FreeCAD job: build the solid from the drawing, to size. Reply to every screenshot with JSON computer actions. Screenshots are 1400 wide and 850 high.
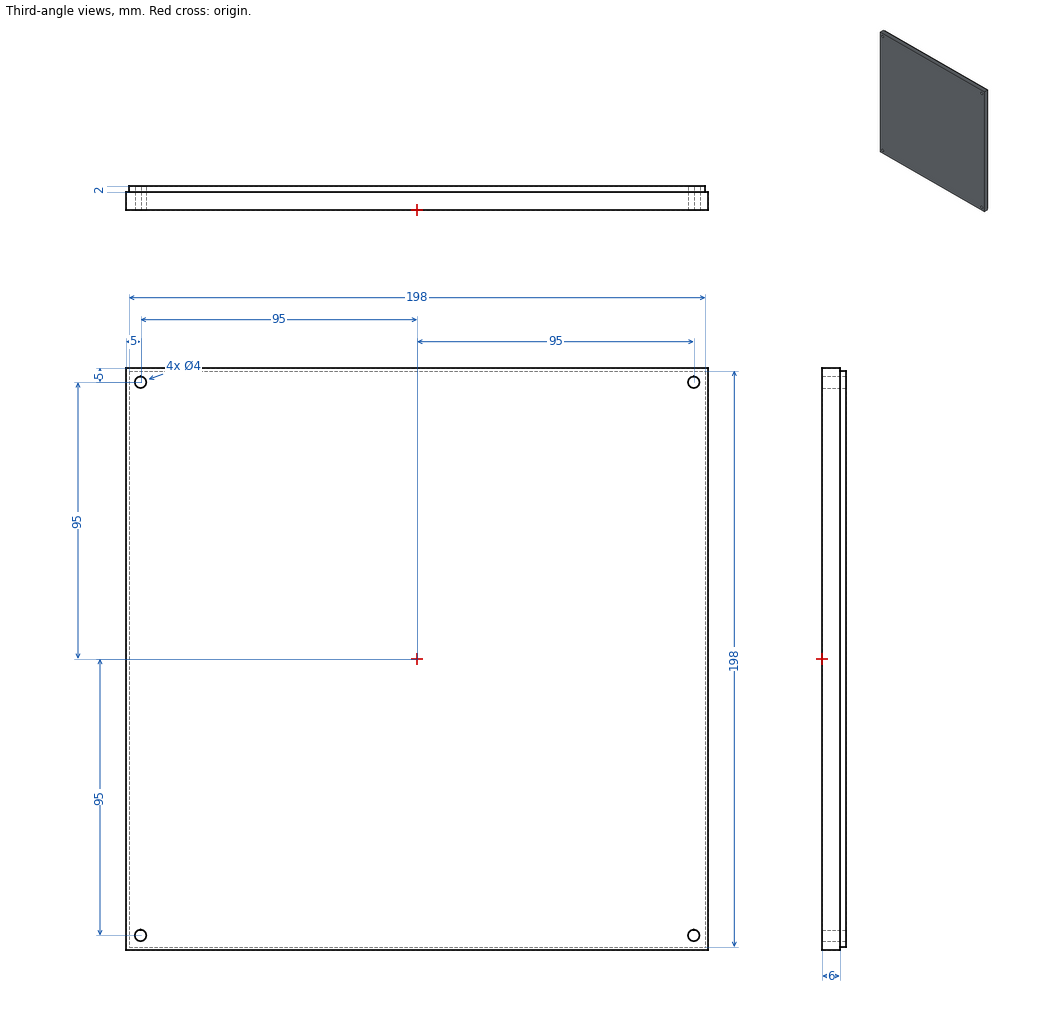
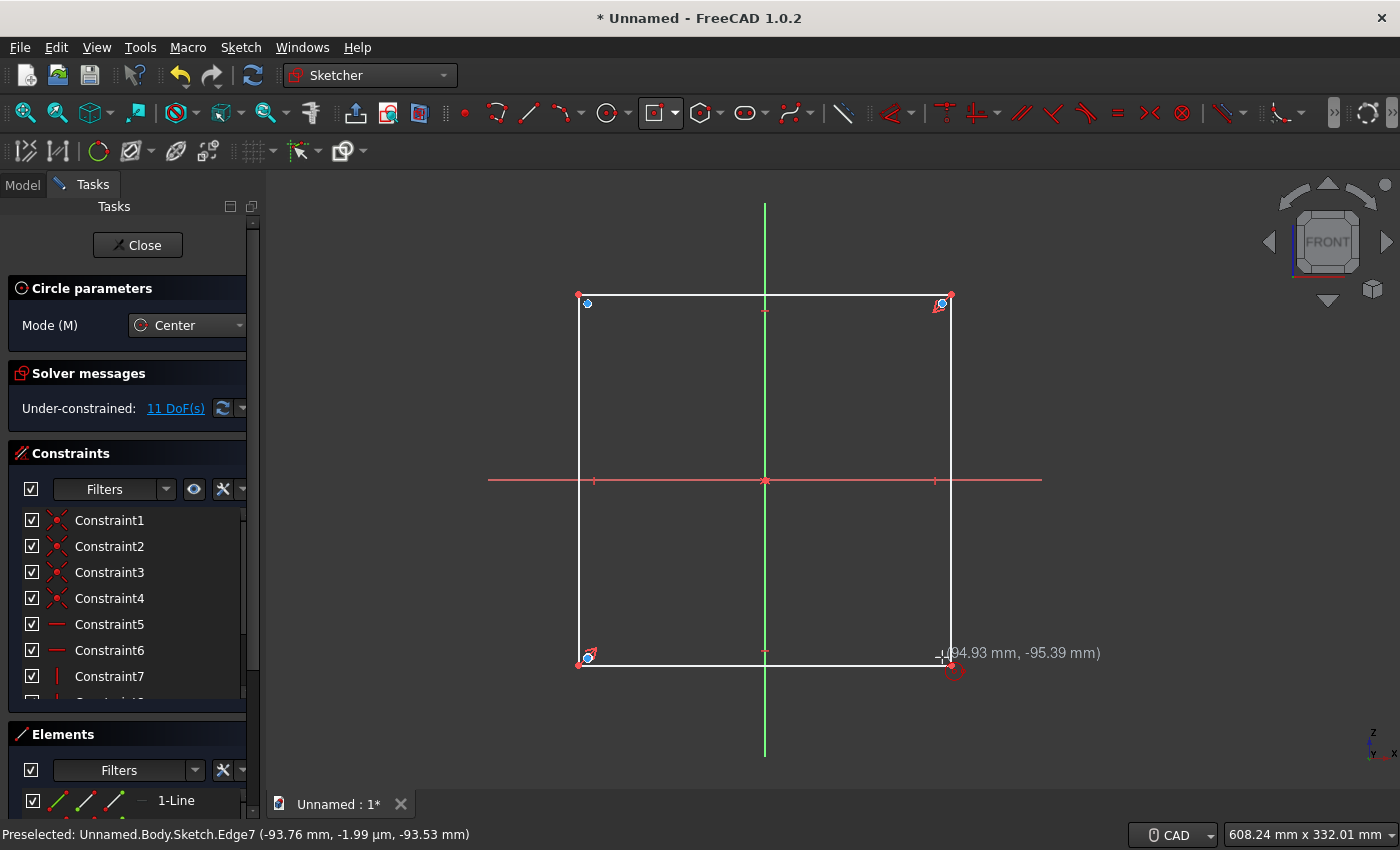
{"action": "scroll", "coordinate": [942, 657], "scroll_direction": "up", "scroll_amount": 3}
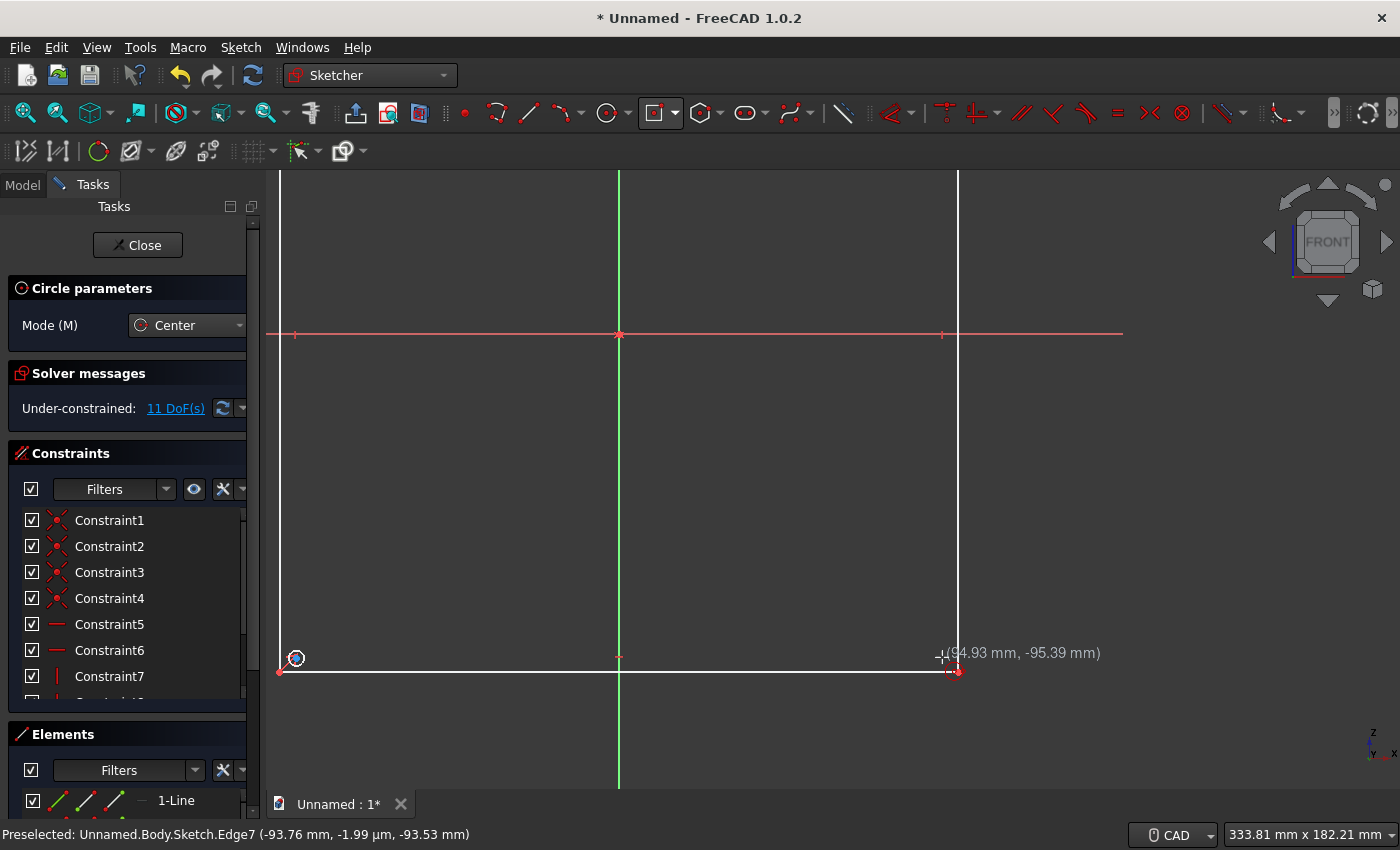
{"action": "left_click", "coordinate": [942, 657]}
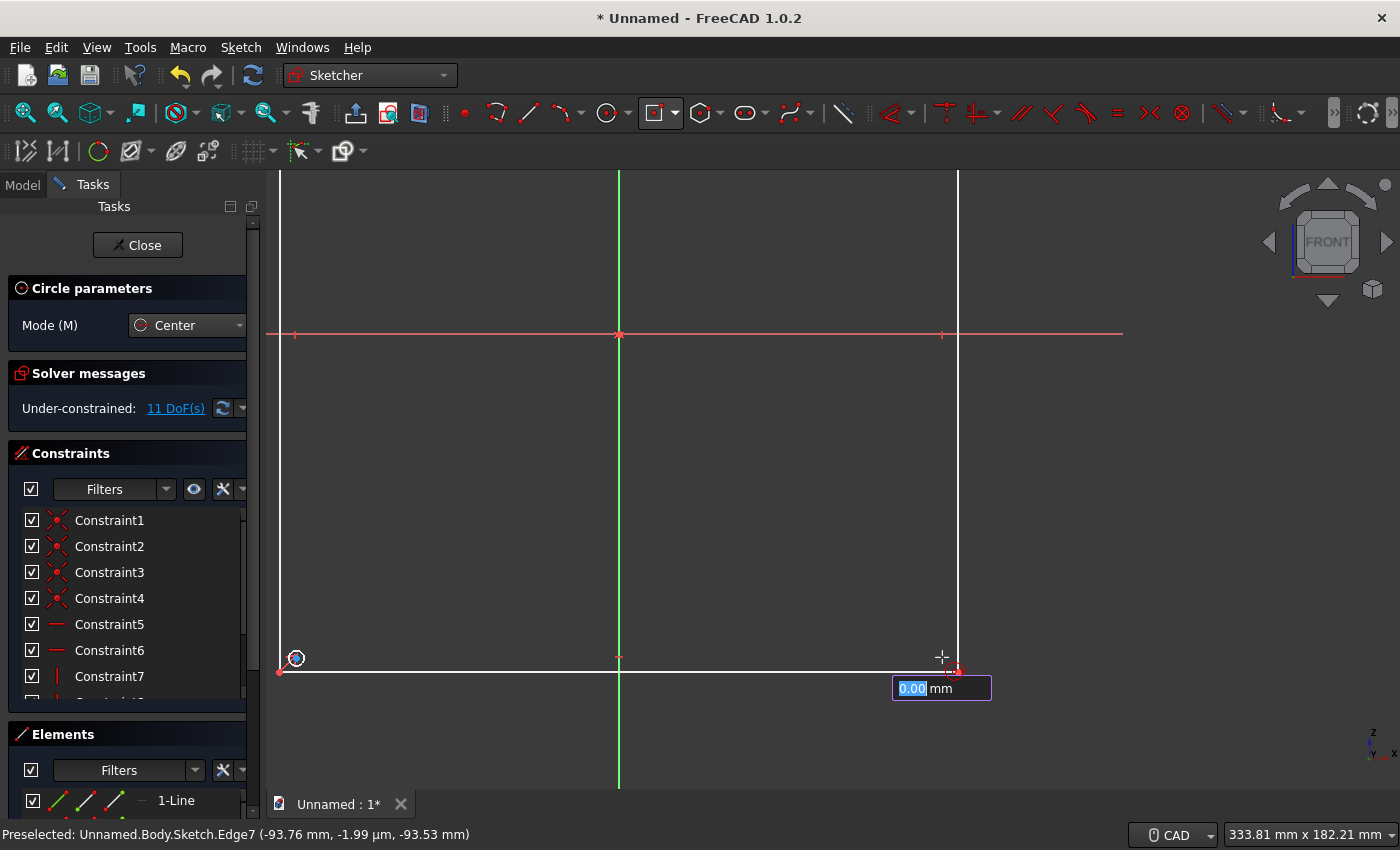
{"action": "scroll", "coordinate": [937, 652], "scroll_direction": "up", "scroll_amount": 5}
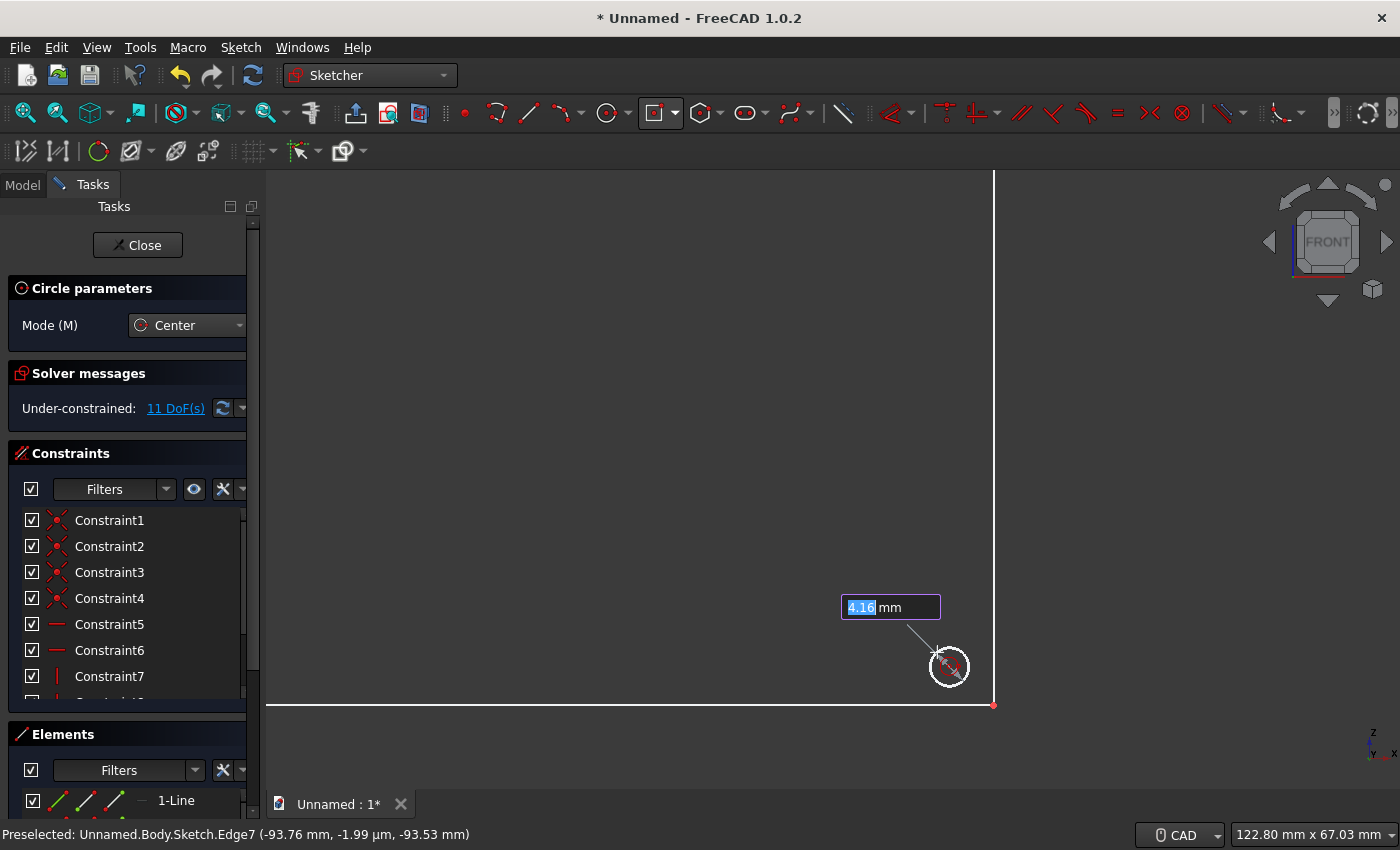
{"action": "left_click", "coordinate": [936, 651]}
{"action": "key", "text": "Escape"}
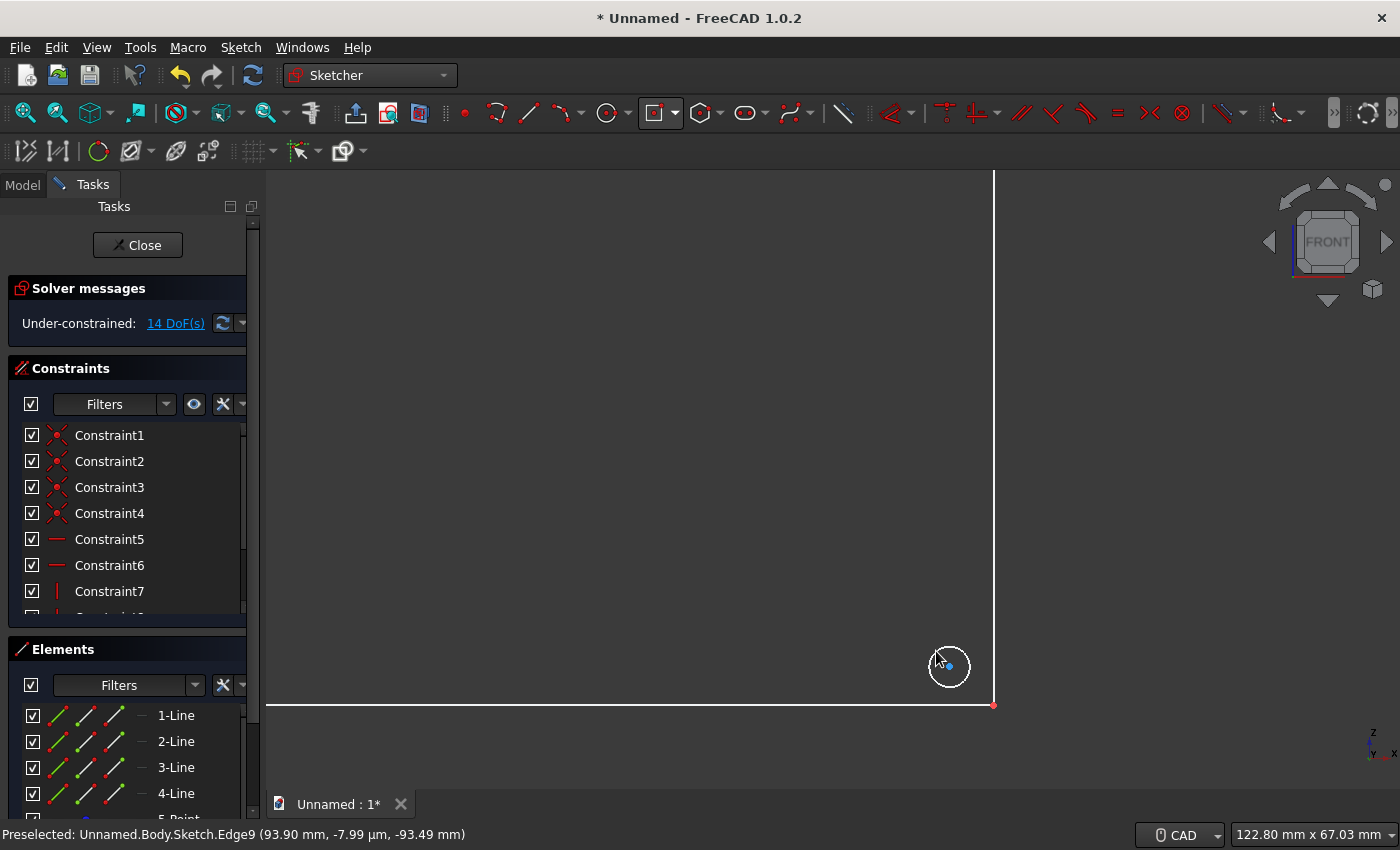
{"action": "scroll", "coordinate": [940, 655], "scroll_direction": "down", "scroll_amount": 8}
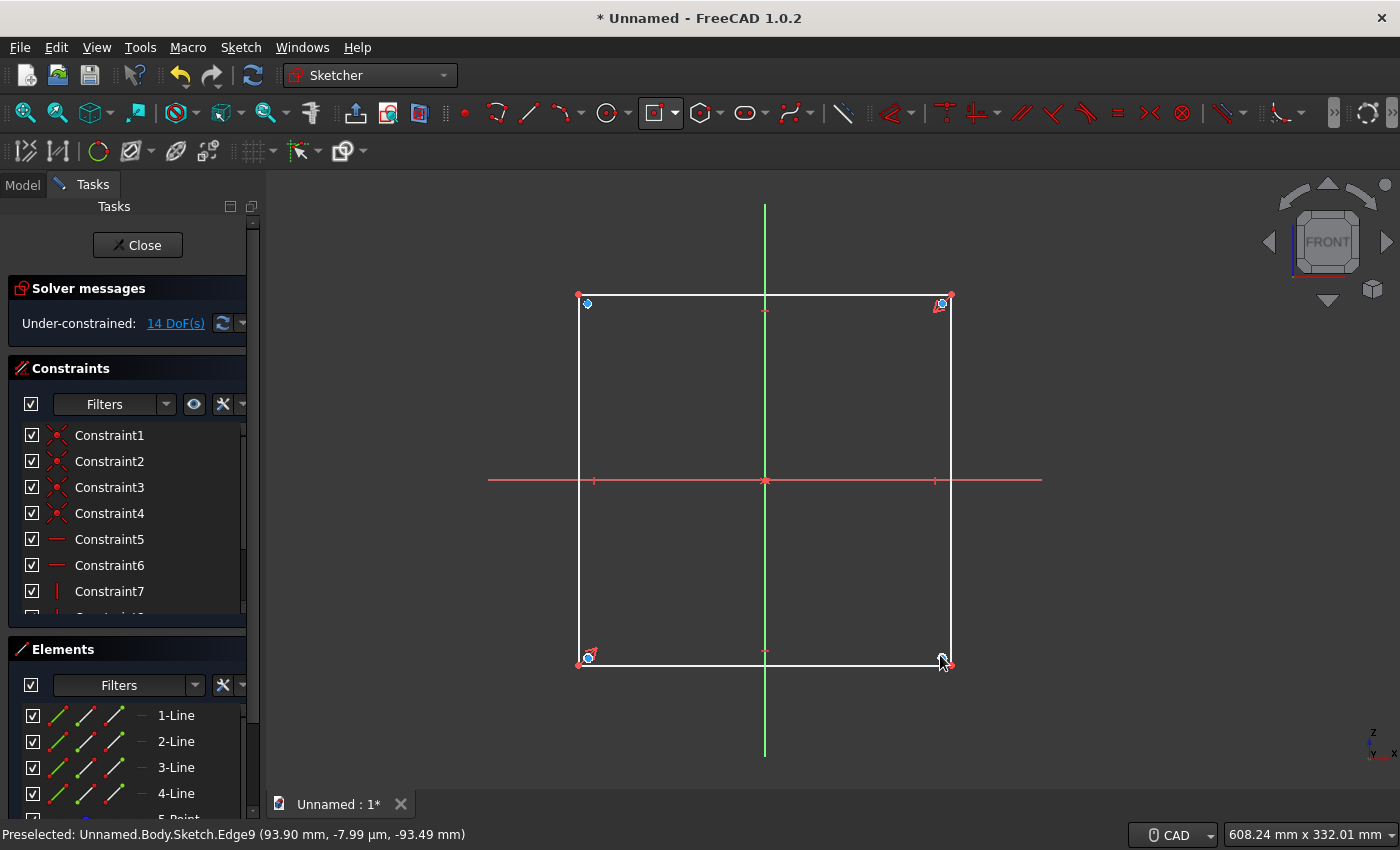
{"action": "scroll", "coordinate": [590, 301], "scroll_direction": "up", "scroll_amount": 7}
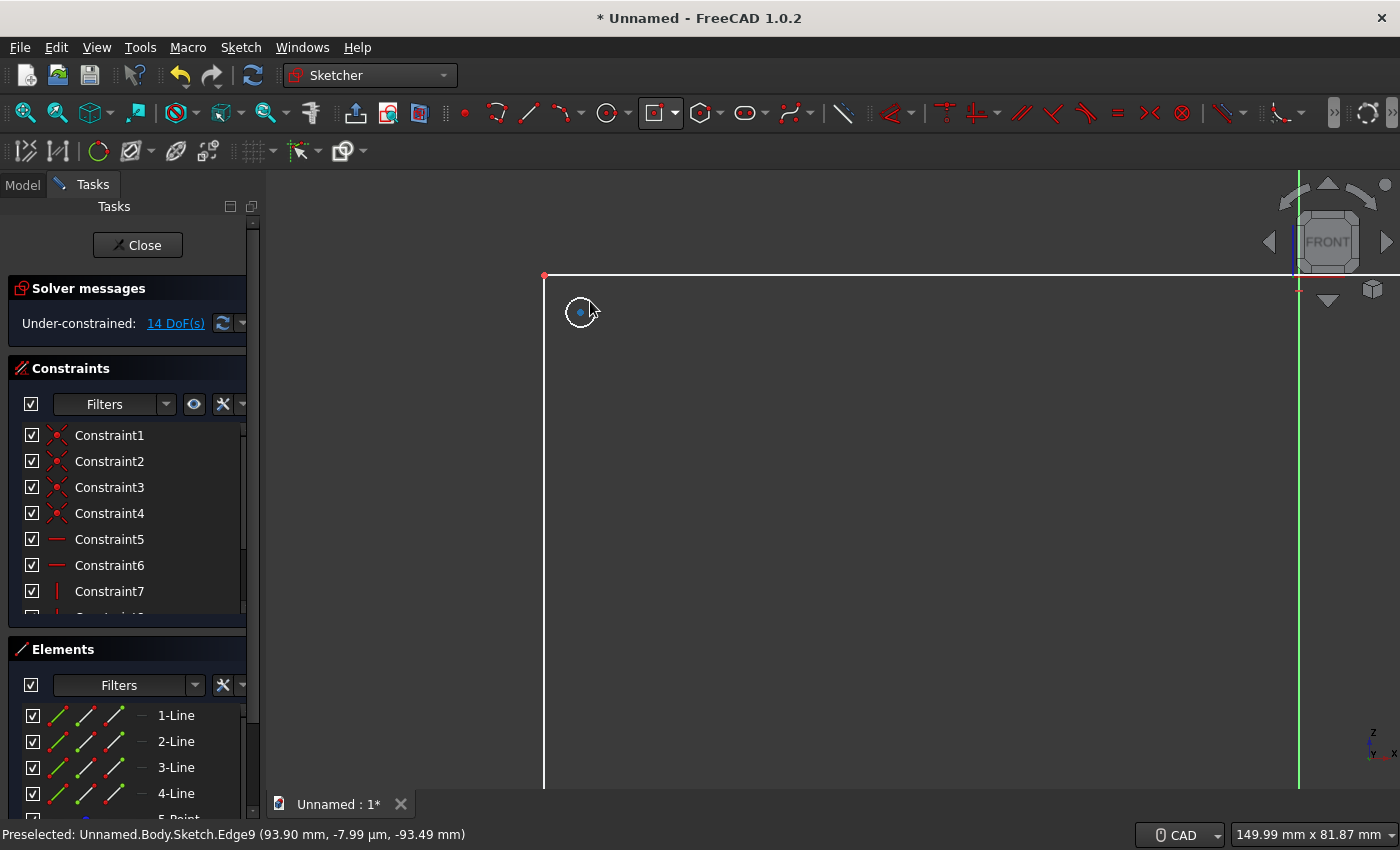
{"action": "left_click", "coordinate": [591, 302]}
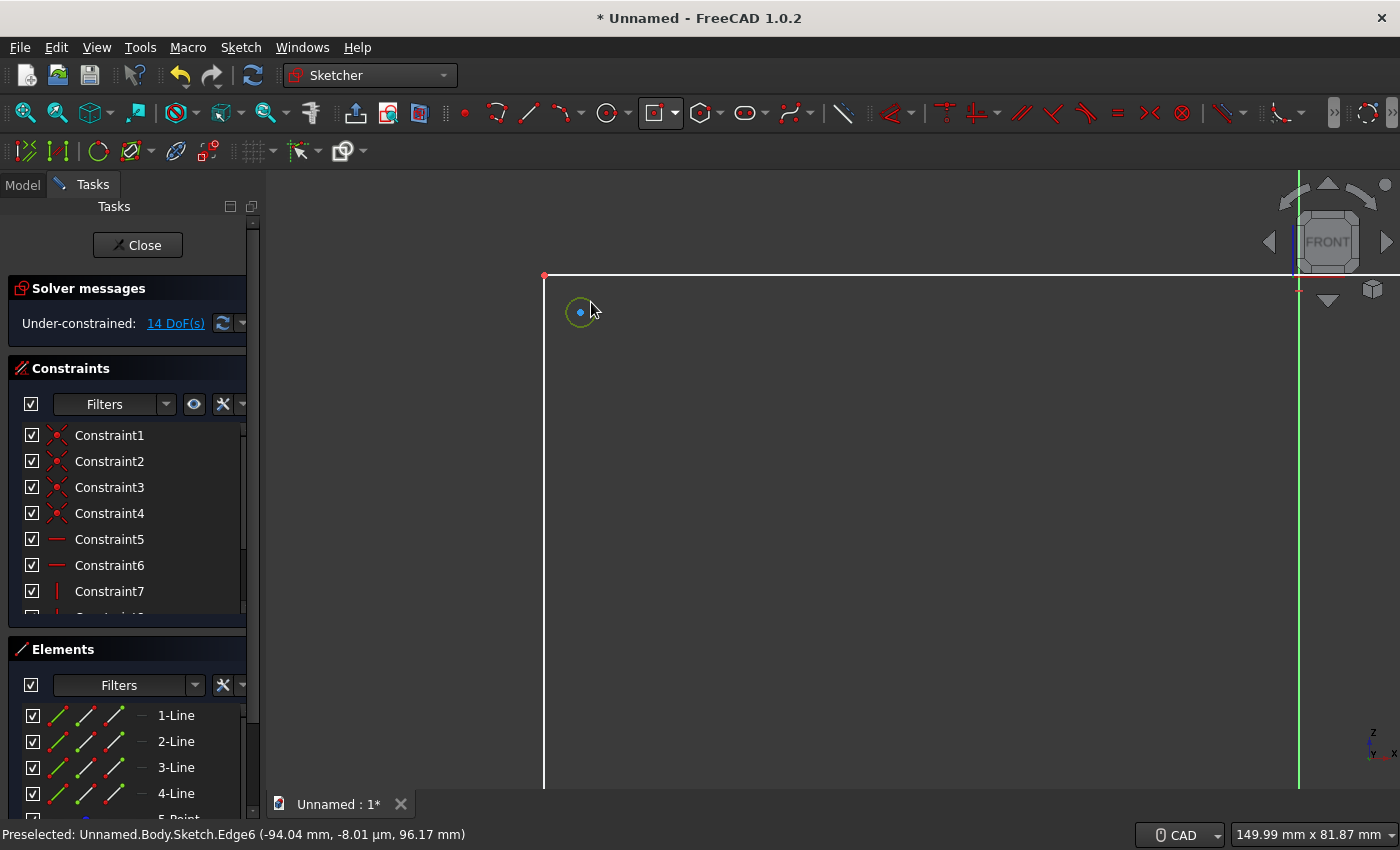
{"action": "scroll", "coordinate": [589, 300], "scroll_direction": "down", "scroll_amount": 7}